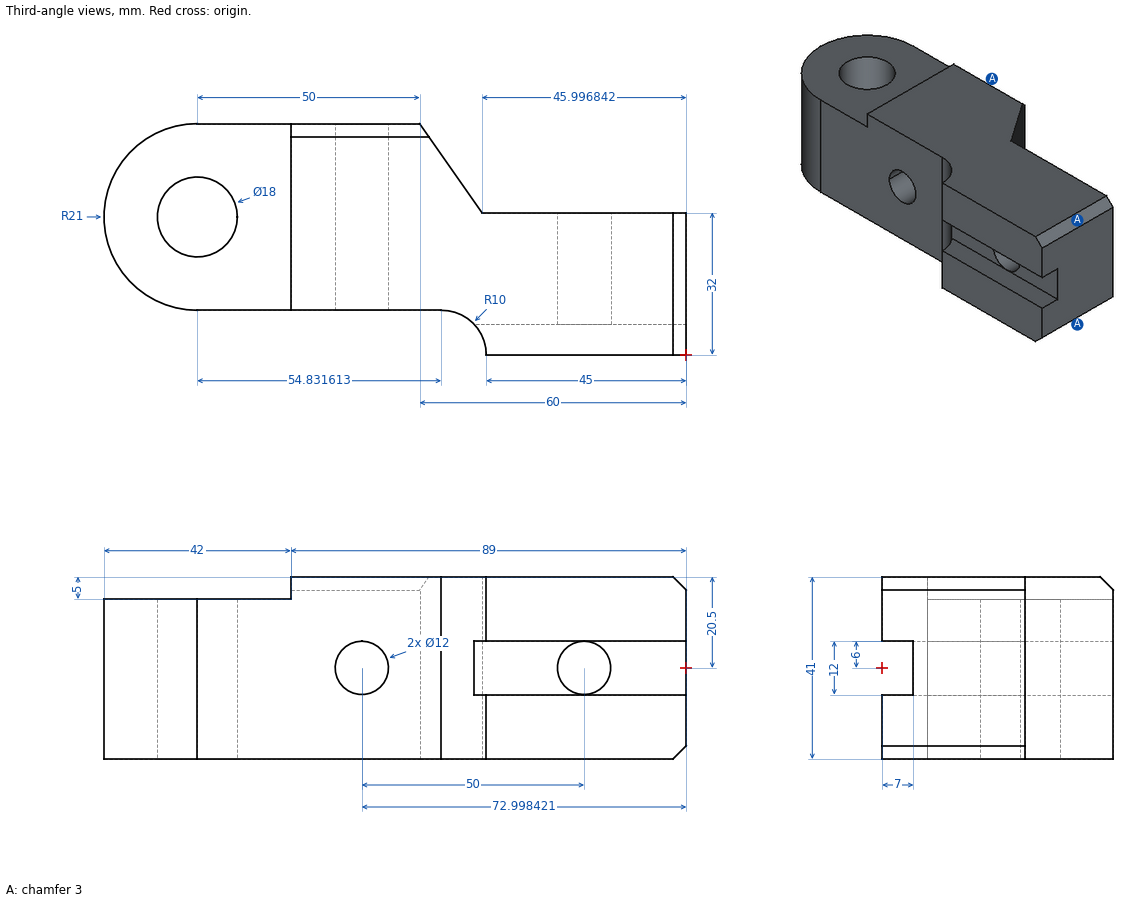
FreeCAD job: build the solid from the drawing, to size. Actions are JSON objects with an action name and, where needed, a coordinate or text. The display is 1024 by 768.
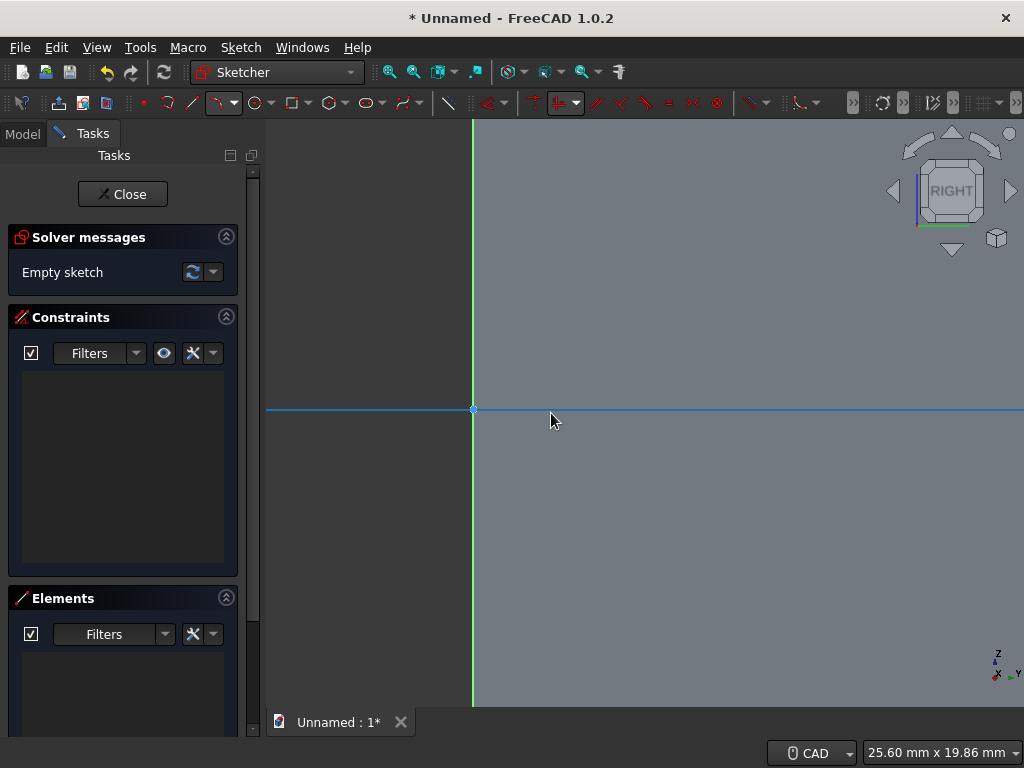
{"action": "left_click", "coordinate": [292, 104]}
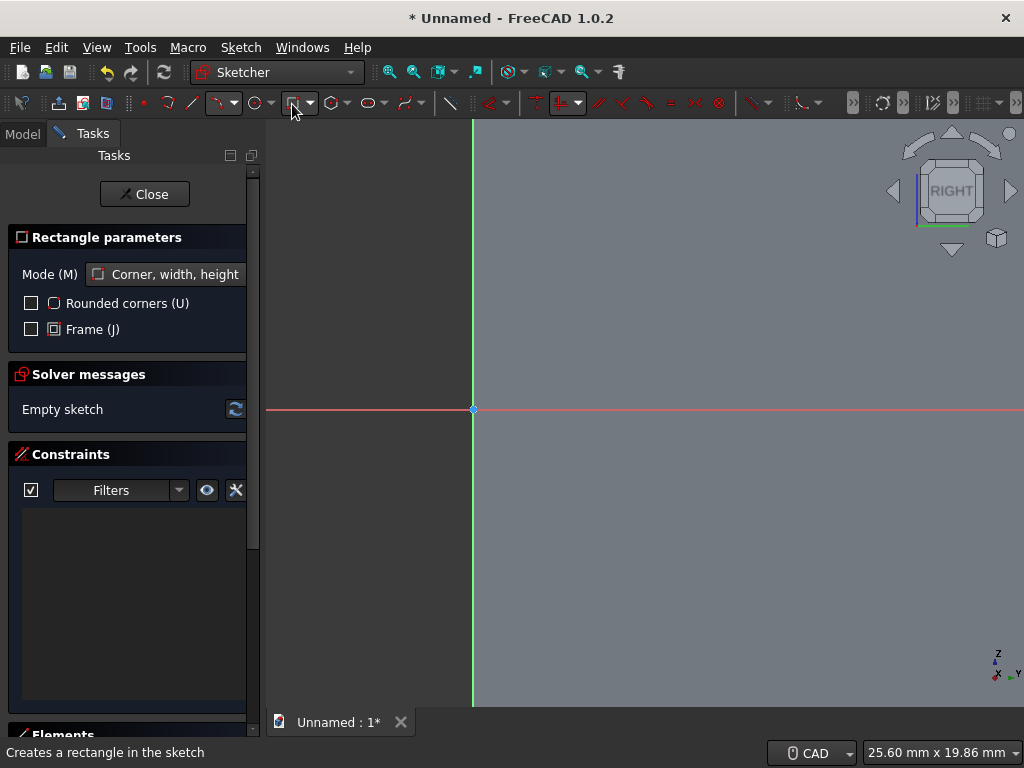
{"action": "left_click", "coordinate": [473, 232]}
{"action": "left_click", "coordinate": [681, 587]}
{"action": "key", "text": "Escape"}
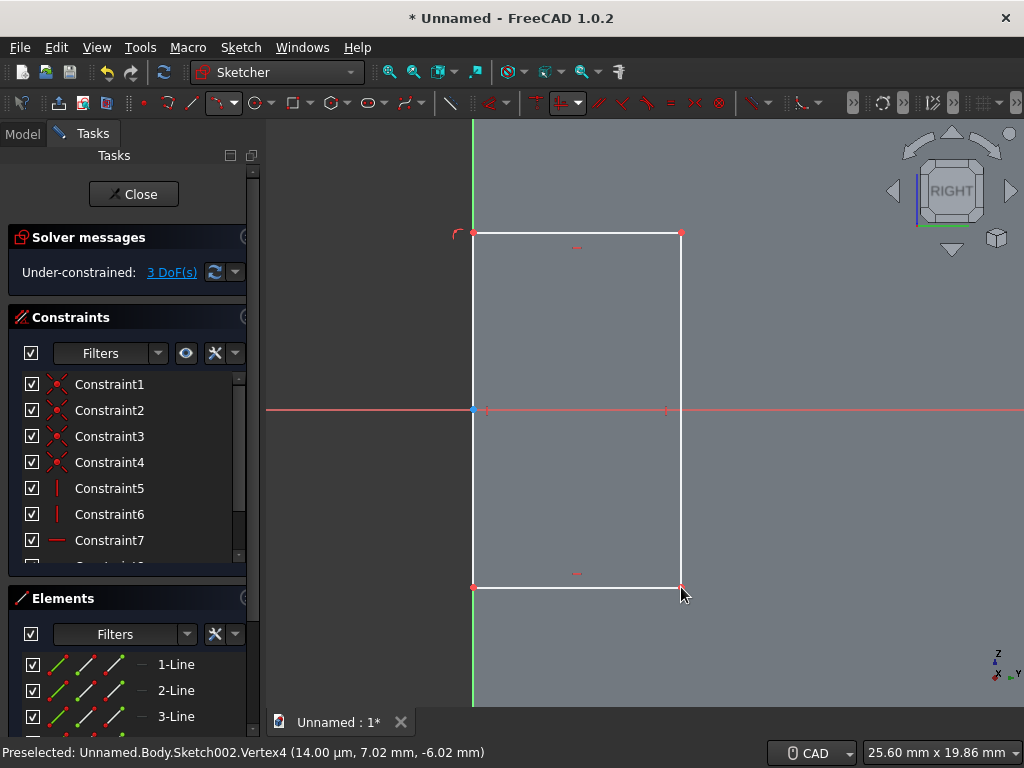
{"action": "left_click", "coordinate": [490, 104]}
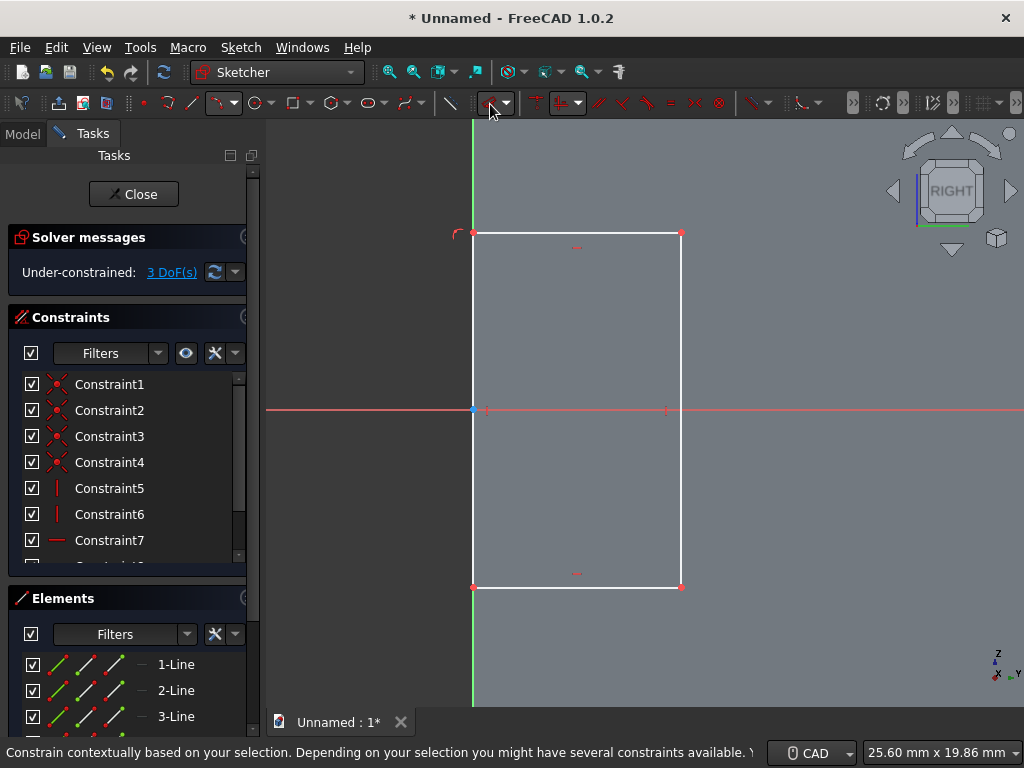
{"action": "left_click", "coordinate": [536, 588]}
{"action": "left_click", "coordinate": [577, 622]}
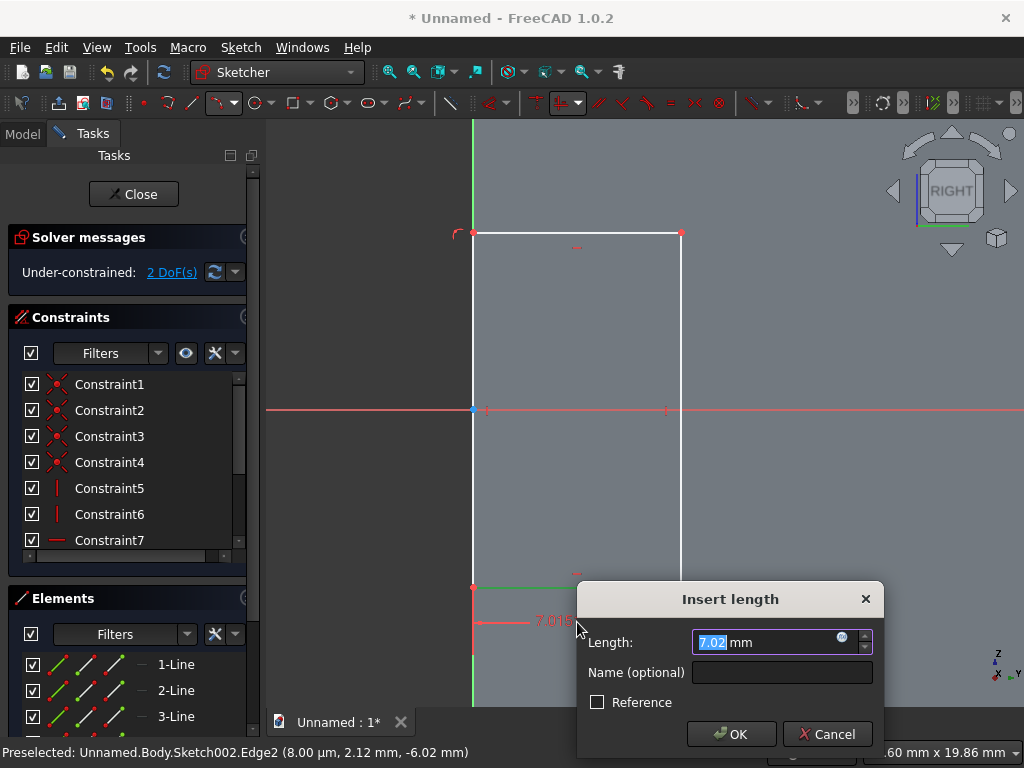
{"action": "type", "text": "7"}
{"action": "key", "text": "Return"}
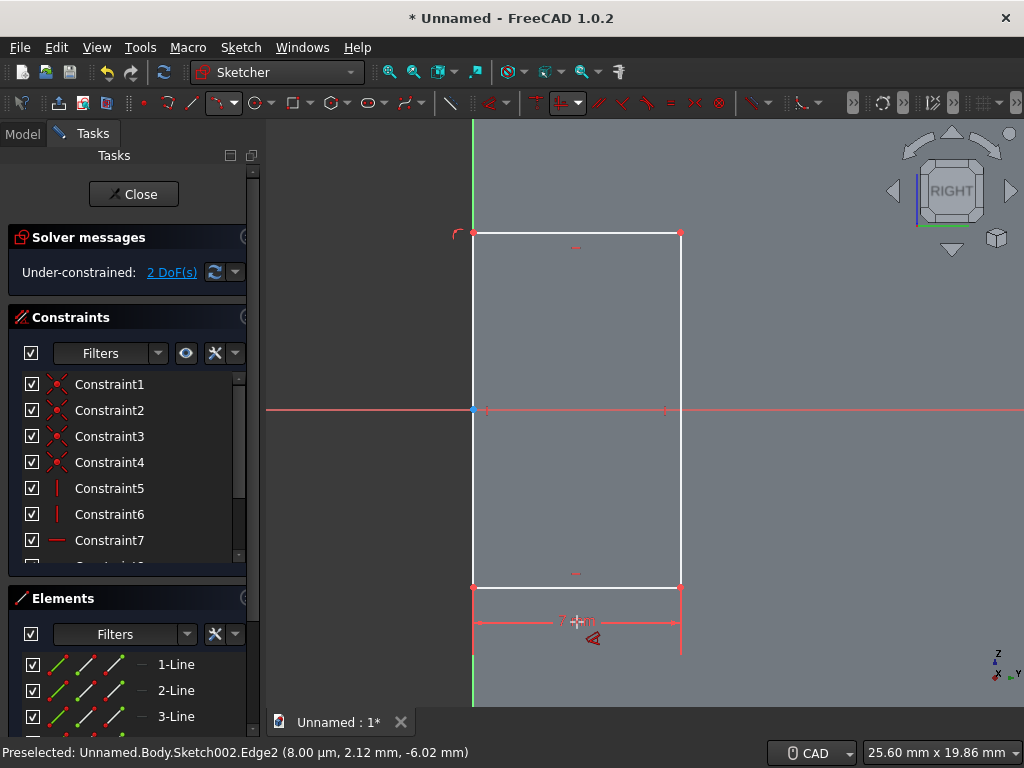
{"action": "left_click", "coordinate": [473, 340]}
{"action": "left_click", "coordinate": [439, 329]}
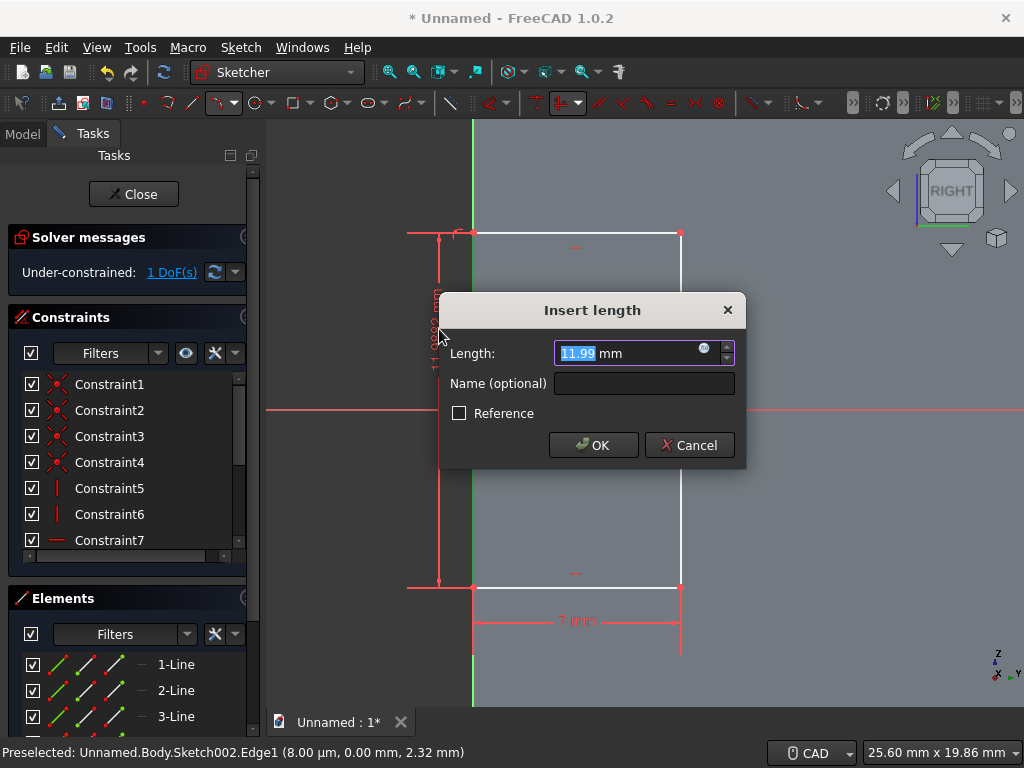
{"action": "type", "text": "12"}
{"action": "key", "text": "Return"}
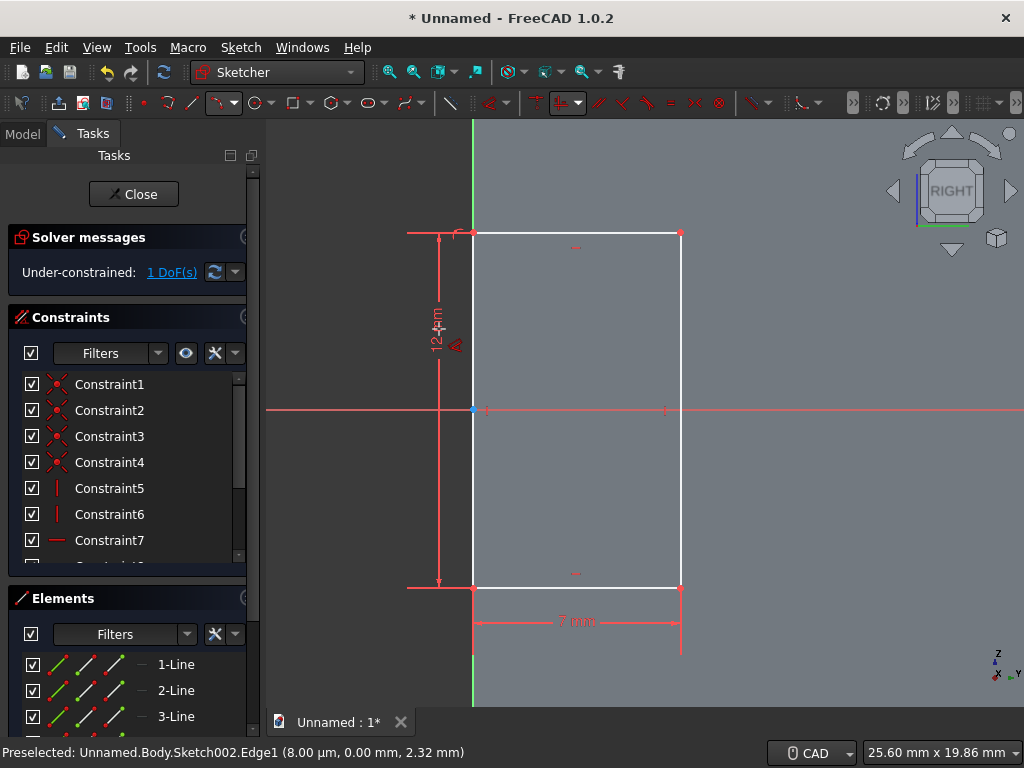
{"action": "left_click", "coordinate": [473, 233]}
{"action": "left_click", "coordinate": [439, 281]}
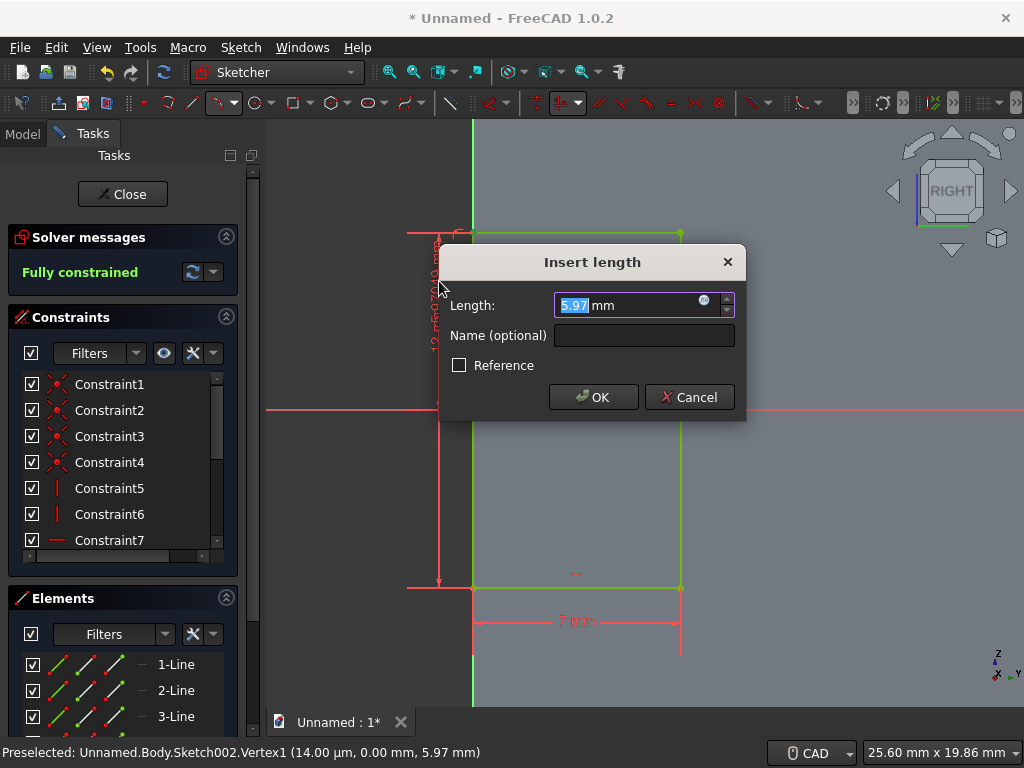
{"action": "type", "text": "6"}
{"action": "key", "text": "Return"}
{"action": "key", "text": "Escape"}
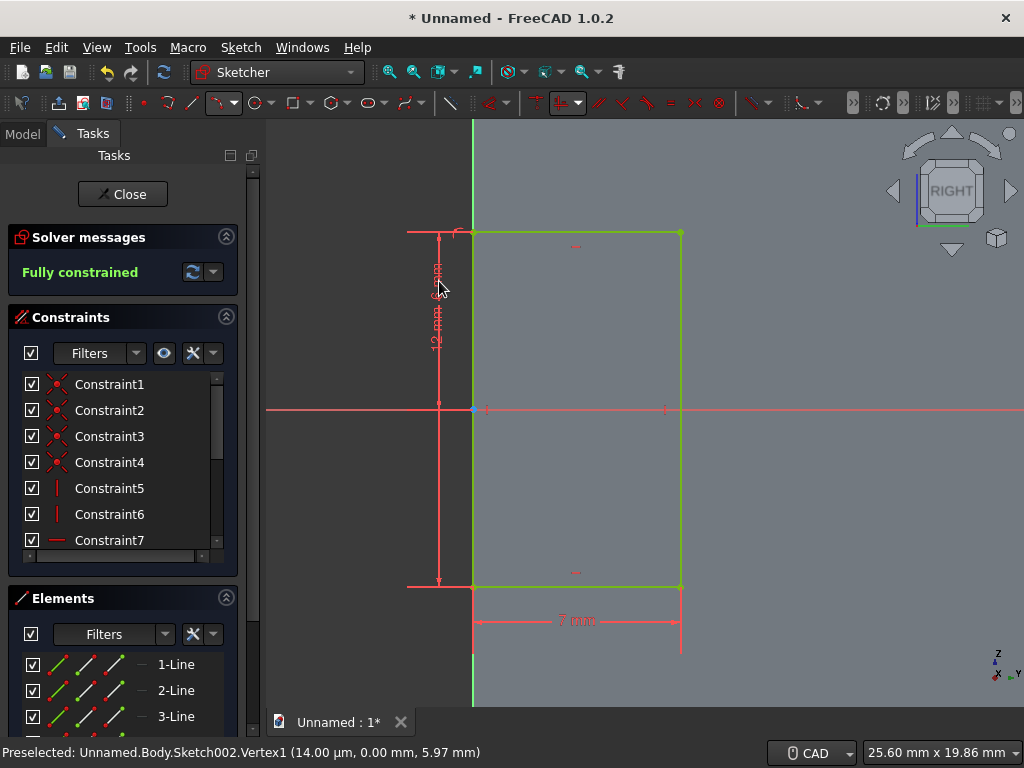
{"action": "left_click", "coordinate": [123, 194]}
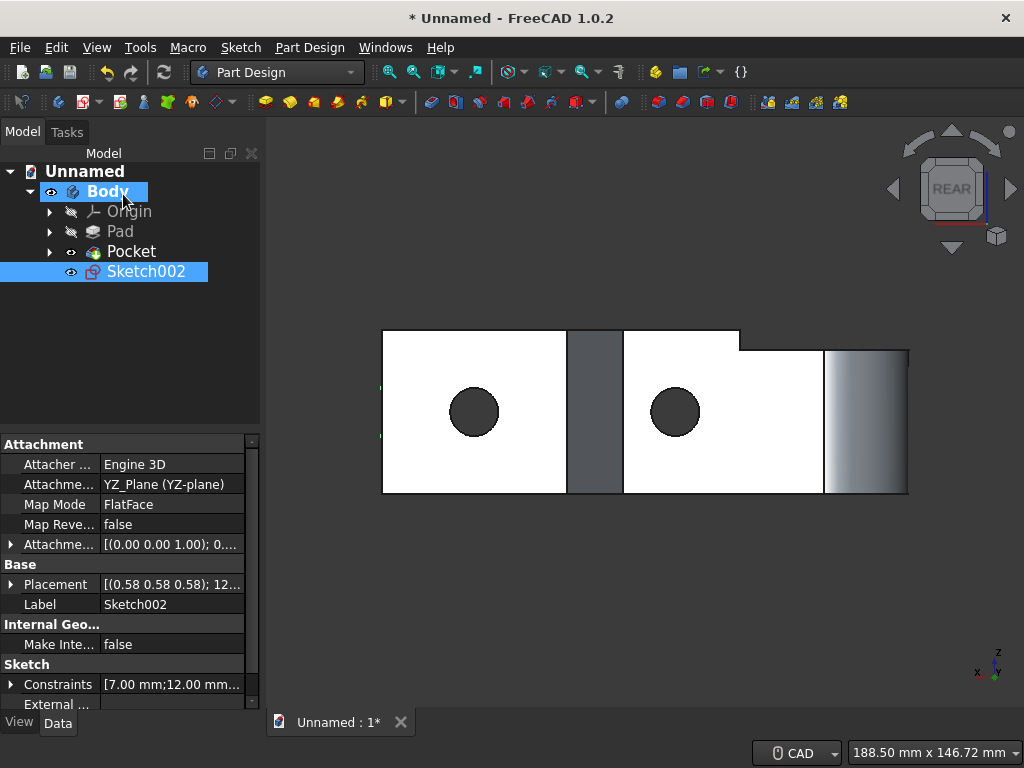
{"action": "left_click", "coordinate": [432, 102]}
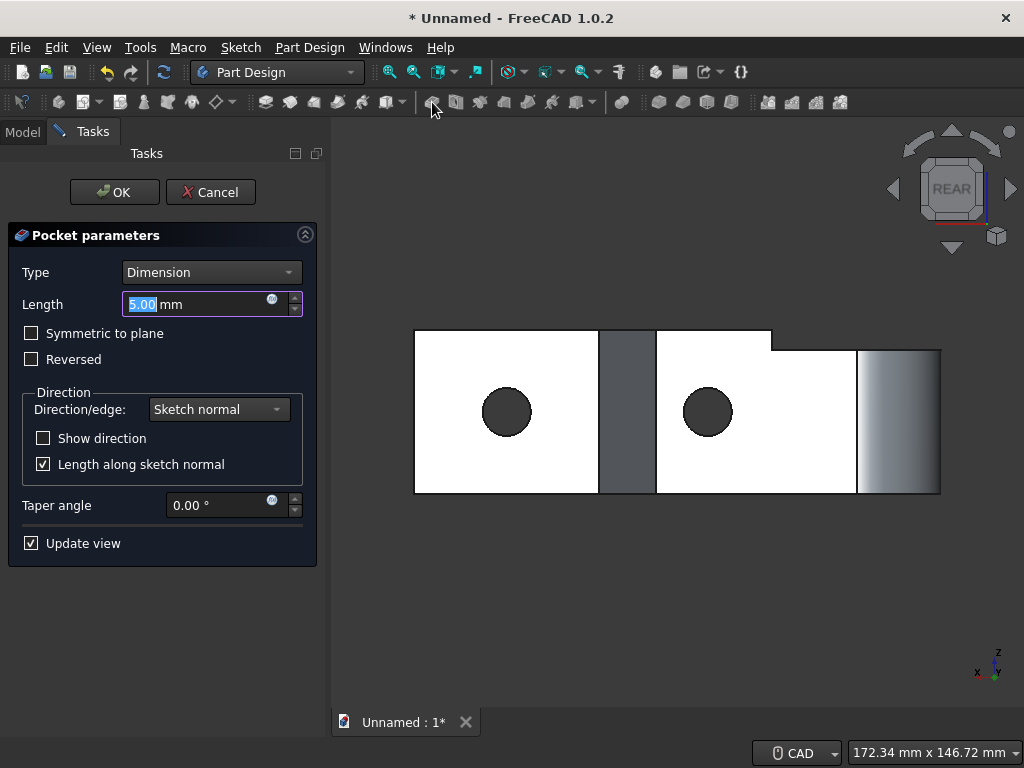
{"action": "left_click", "coordinate": [212, 272]}